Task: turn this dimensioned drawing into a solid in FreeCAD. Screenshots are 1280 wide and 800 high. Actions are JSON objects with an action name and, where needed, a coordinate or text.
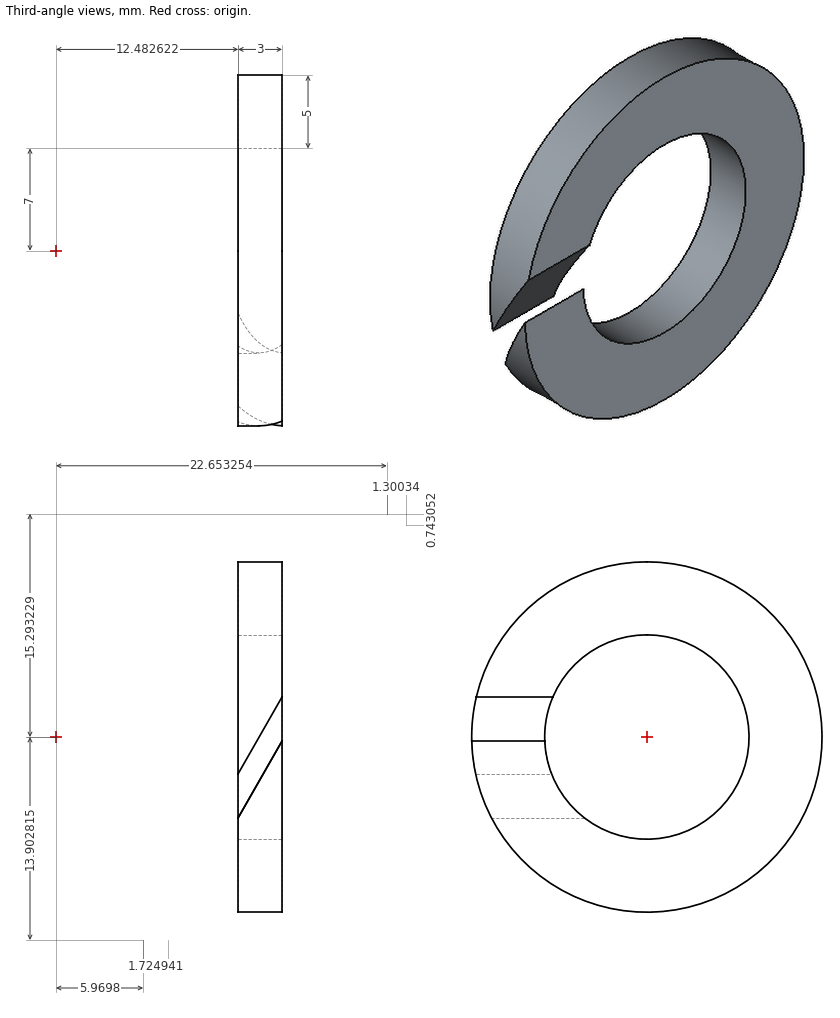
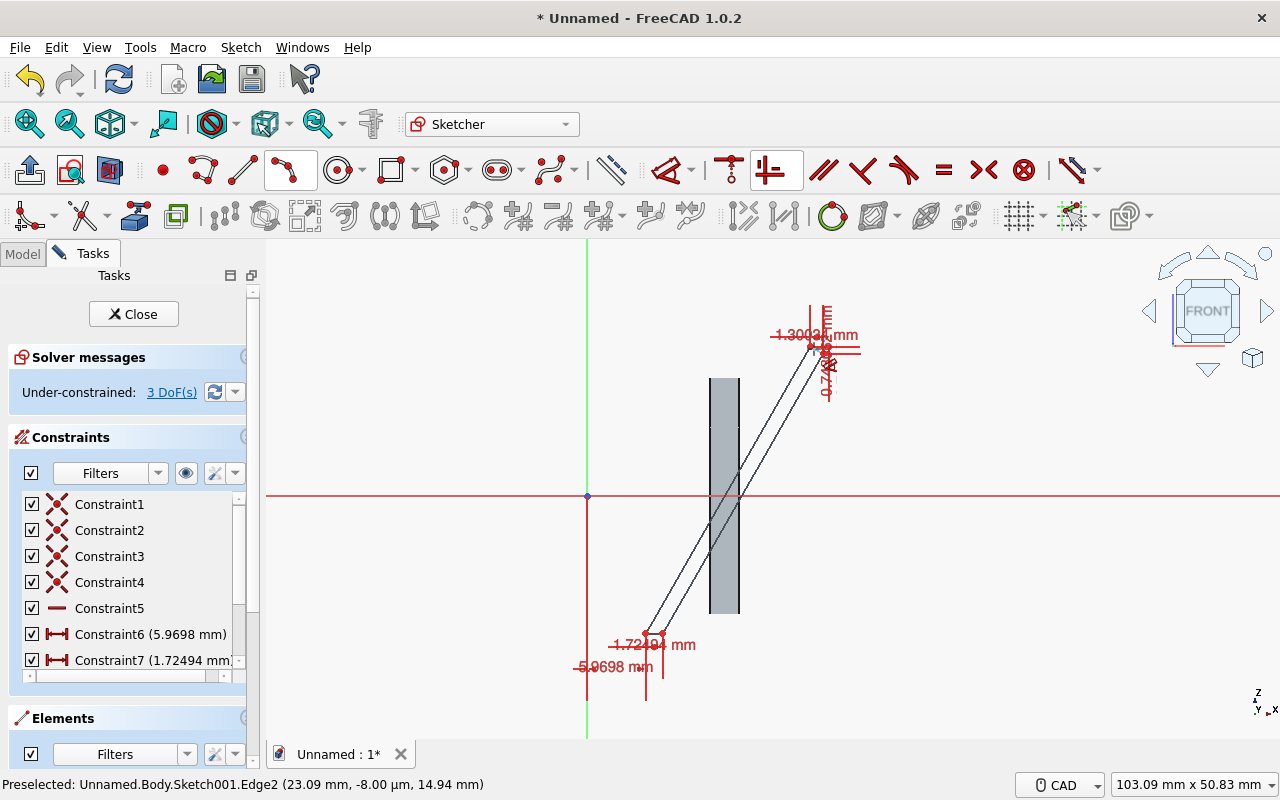
{"action": "left_click", "coordinate": [646, 634]}
{"action": "left_click", "coordinate": [553, 565]}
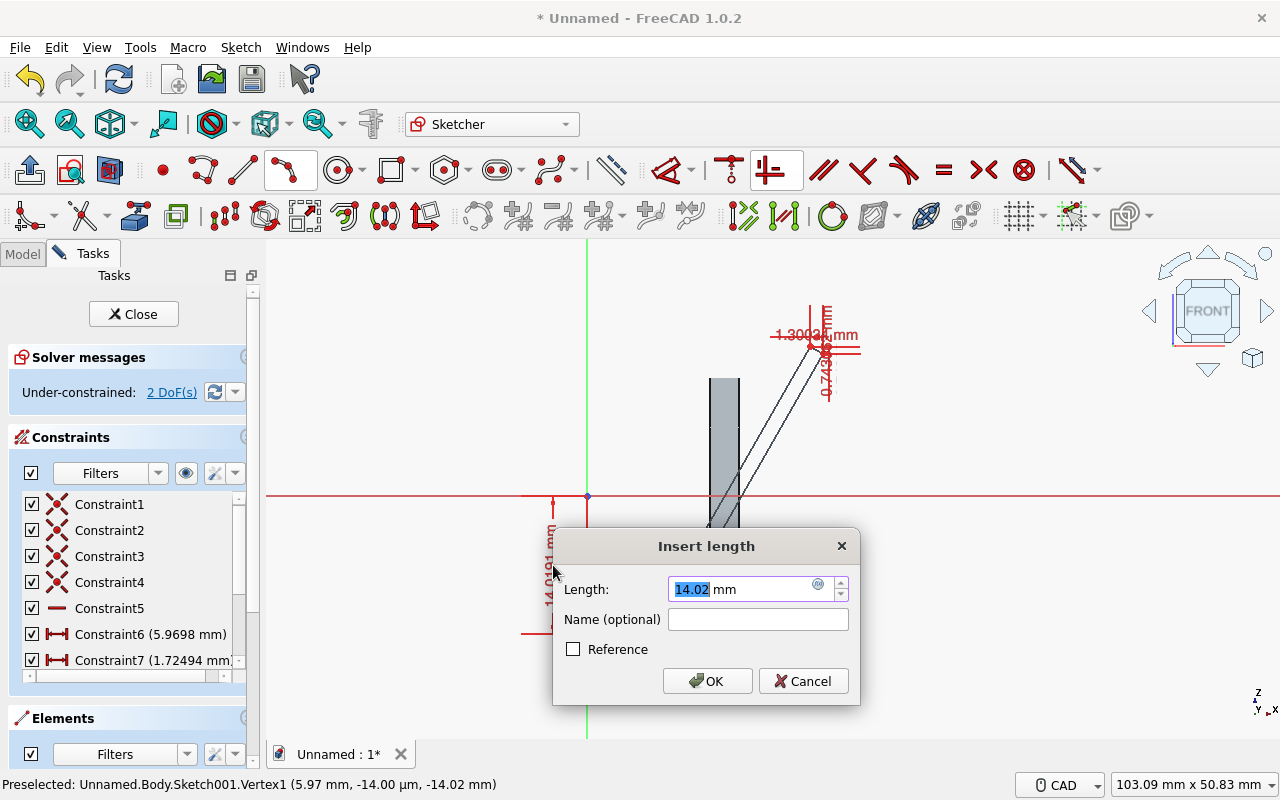
{"action": "type", "text": "13.902815"}
{"action": "key", "text": "Return"}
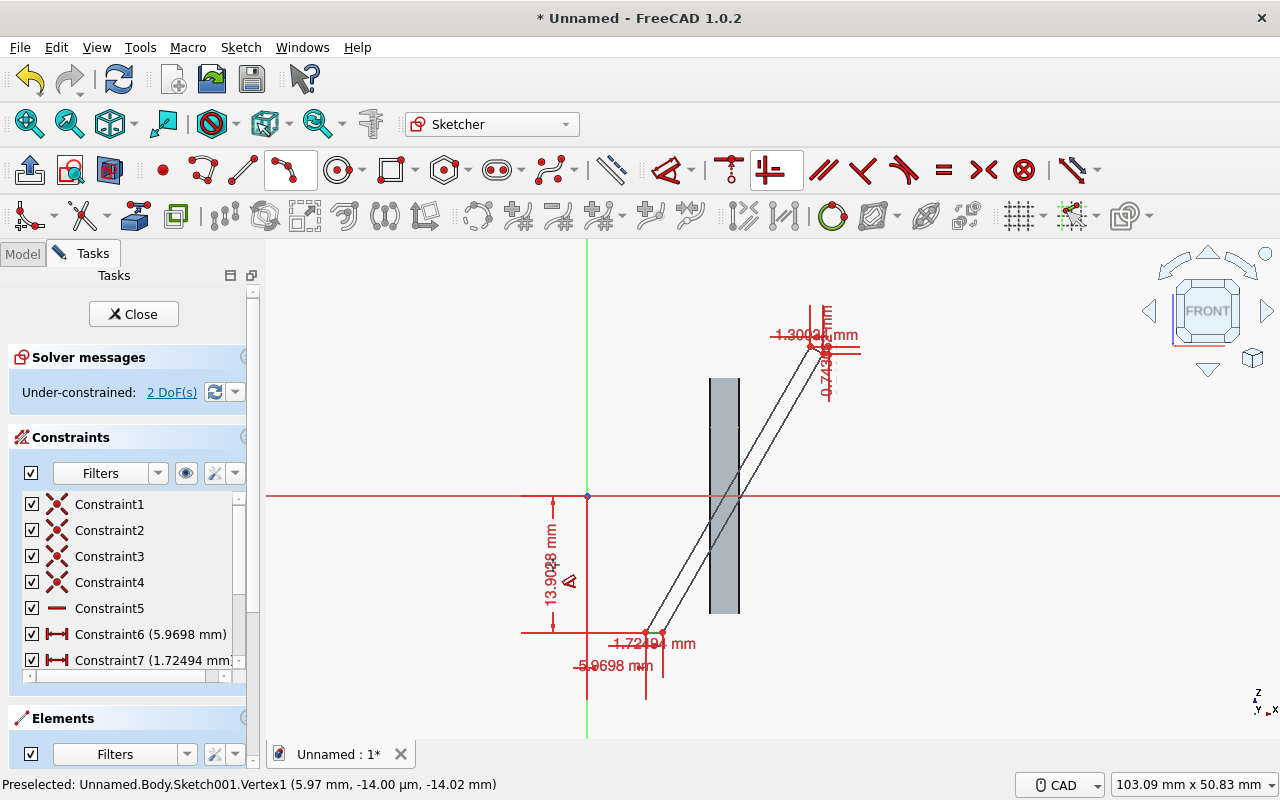
{"action": "left_click", "coordinate": [810, 347]}
{"action": "left_click", "coordinate": [699, 313]}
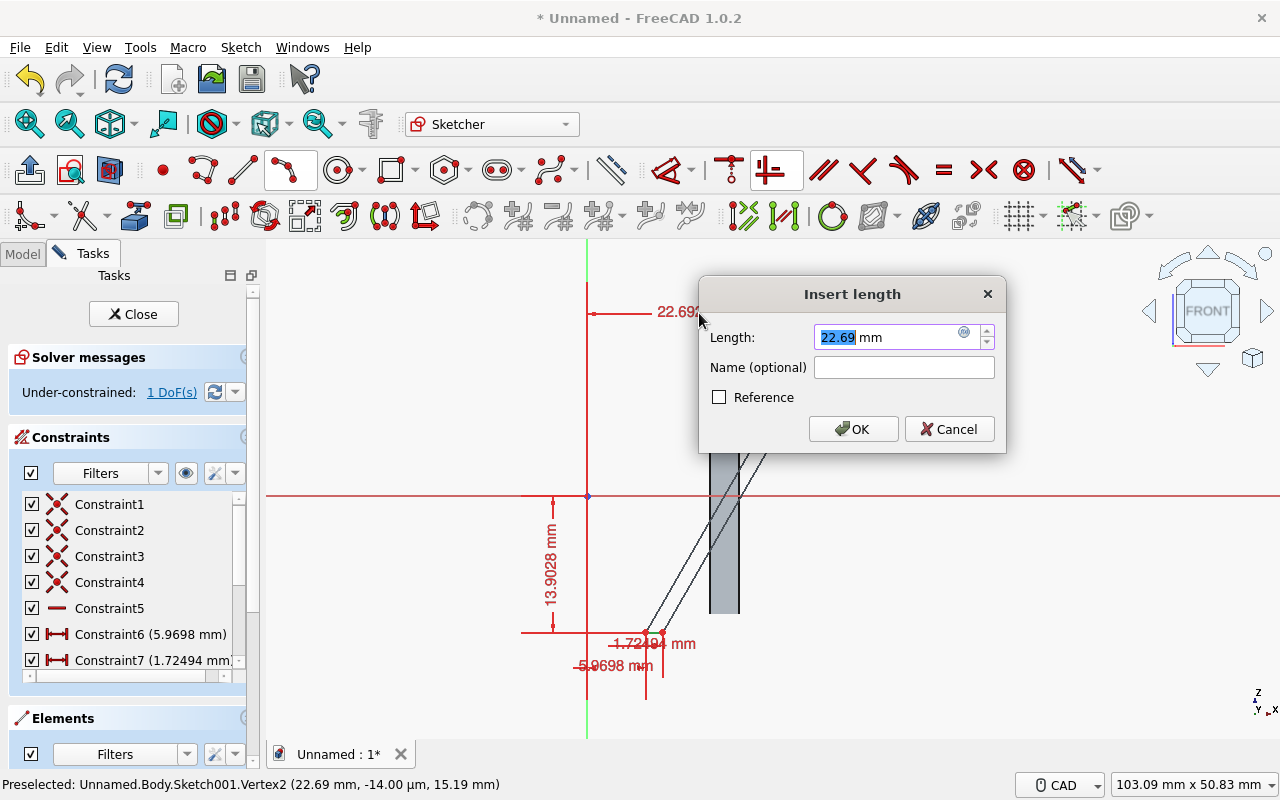
{"action": "type", "text": "22.653254"}
{"action": "key", "text": "Return"}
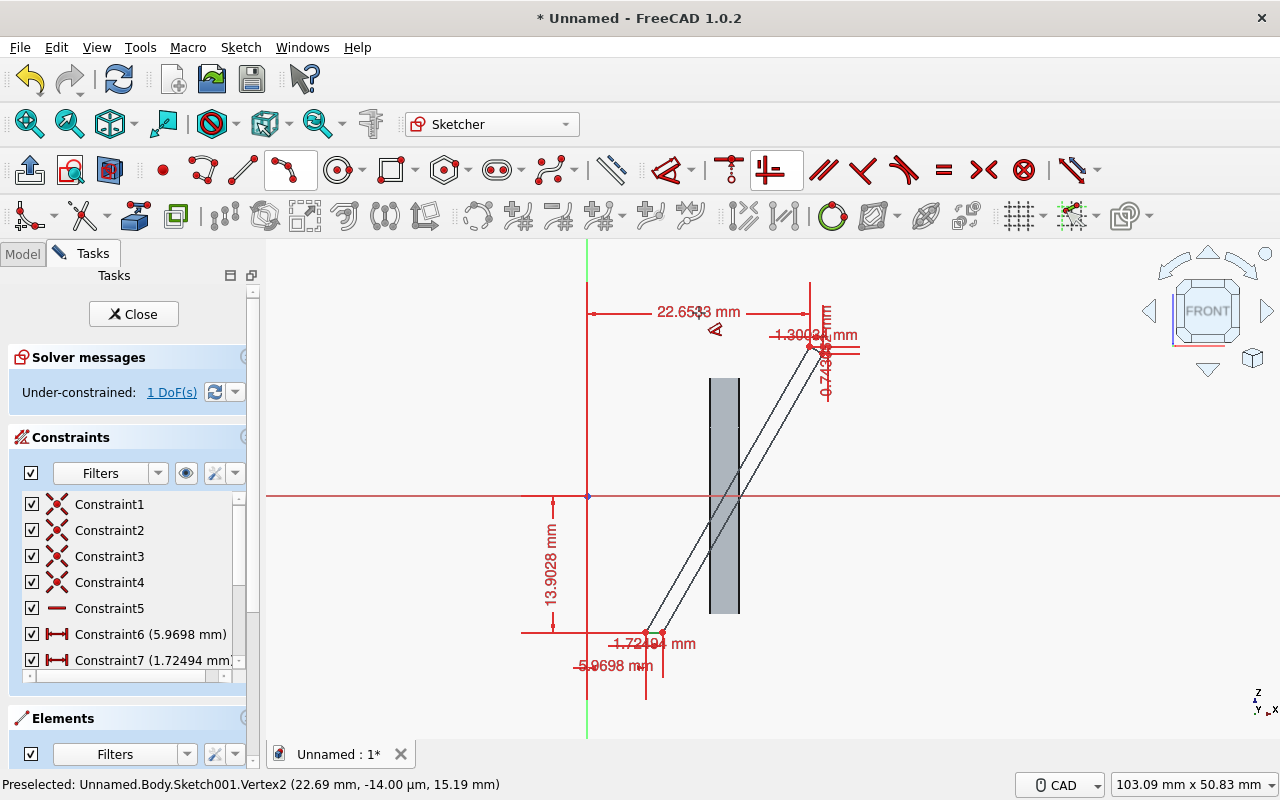
{"action": "left_click", "coordinate": [810, 347]}
{"action": "left_click", "coordinate": [553, 421]}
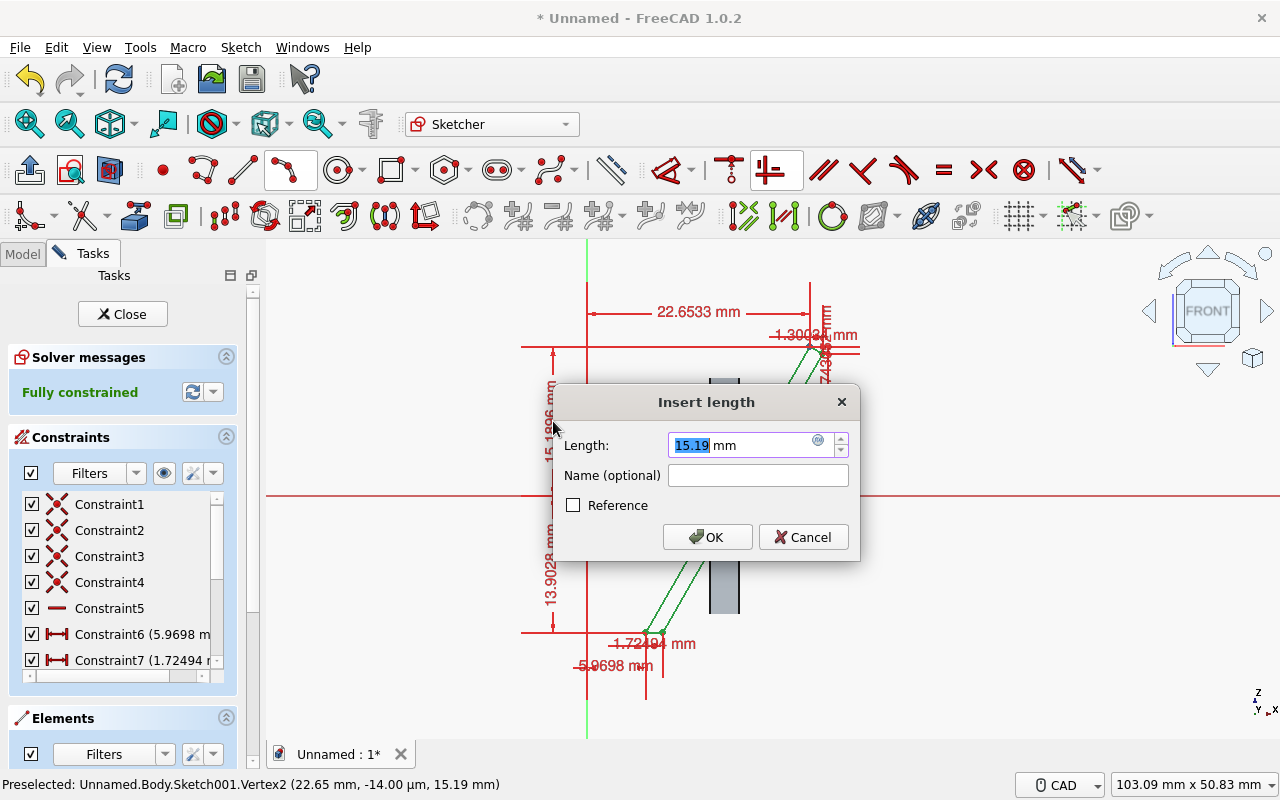
{"action": "type", "text": "15.293229"}
{"action": "key", "text": "Return"}
{"action": "key", "text": "Escape"}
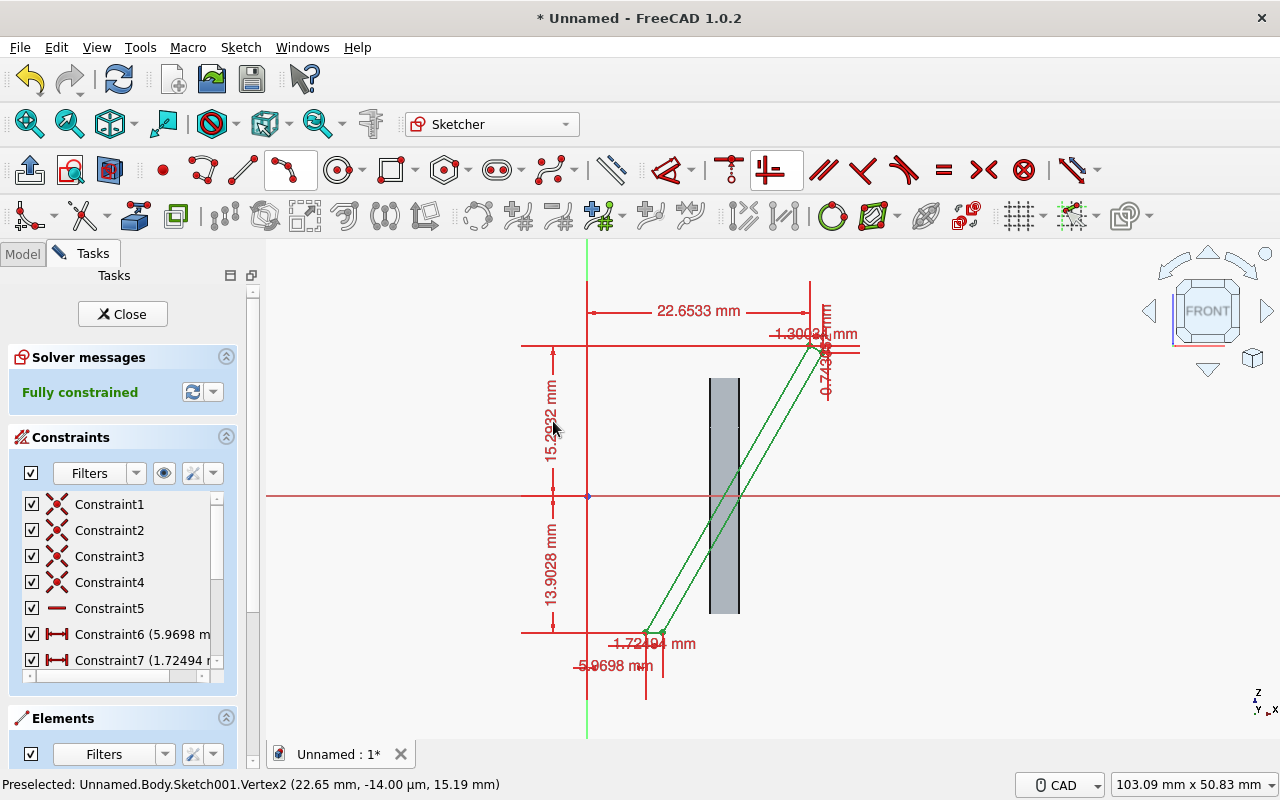
{"action": "left_click", "coordinate": [123, 314]}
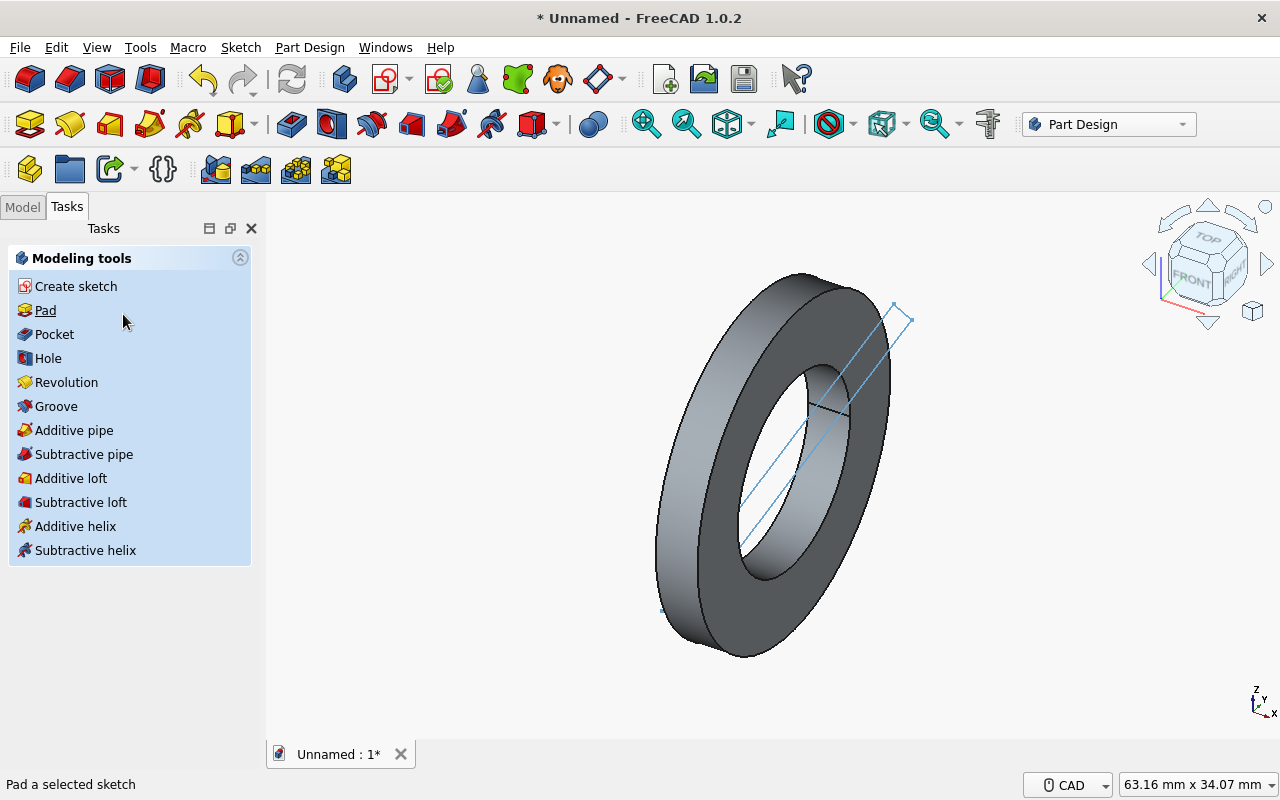
{"action": "left_click", "coordinate": [292, 124]}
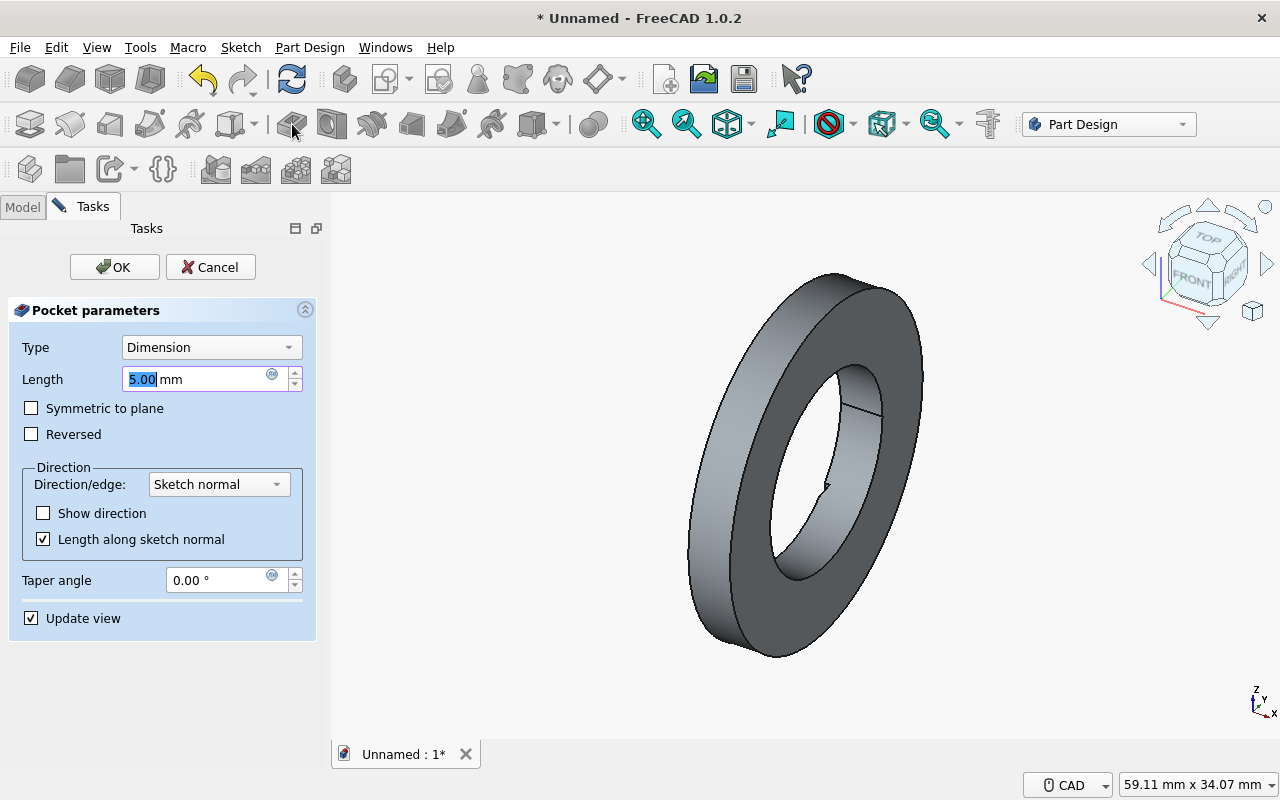
{"action": "left_click", "coordinate": [212, 348]}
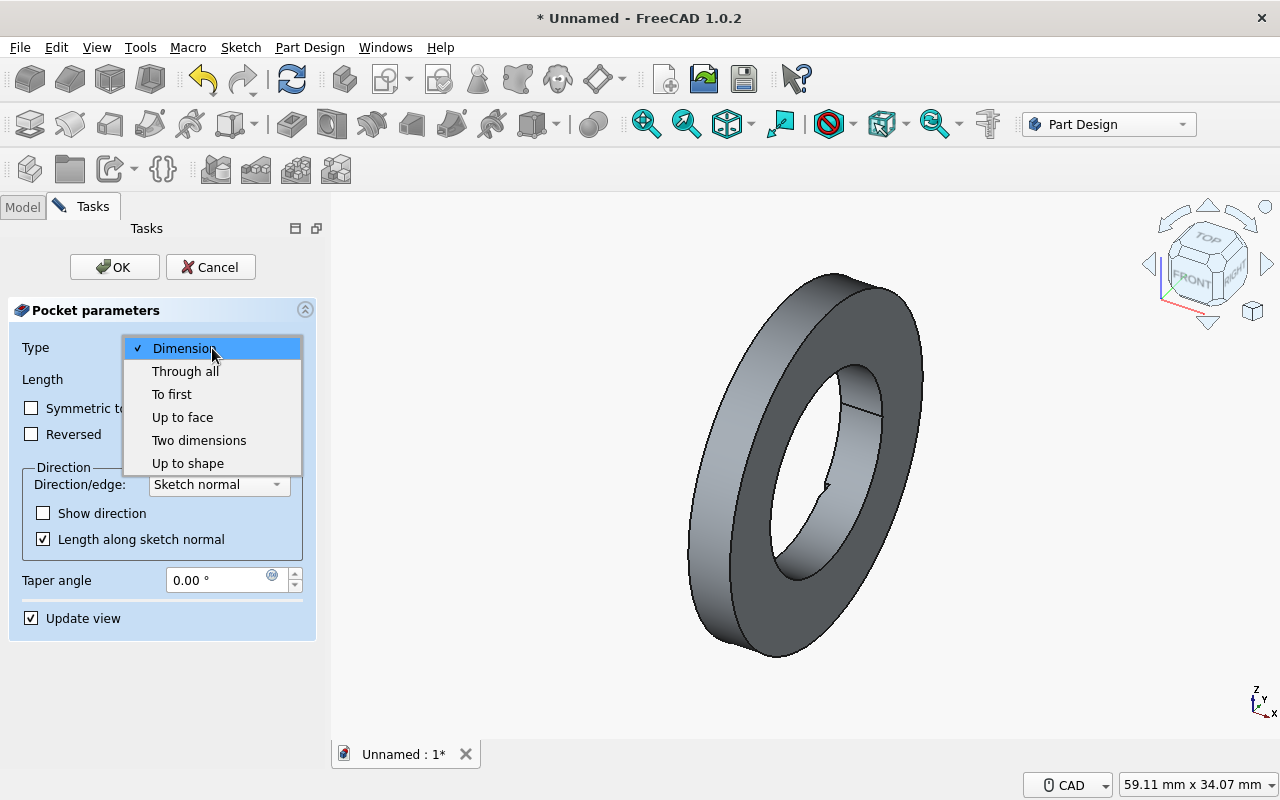
{"action": "left_click", "coordinate": [212, 394]}